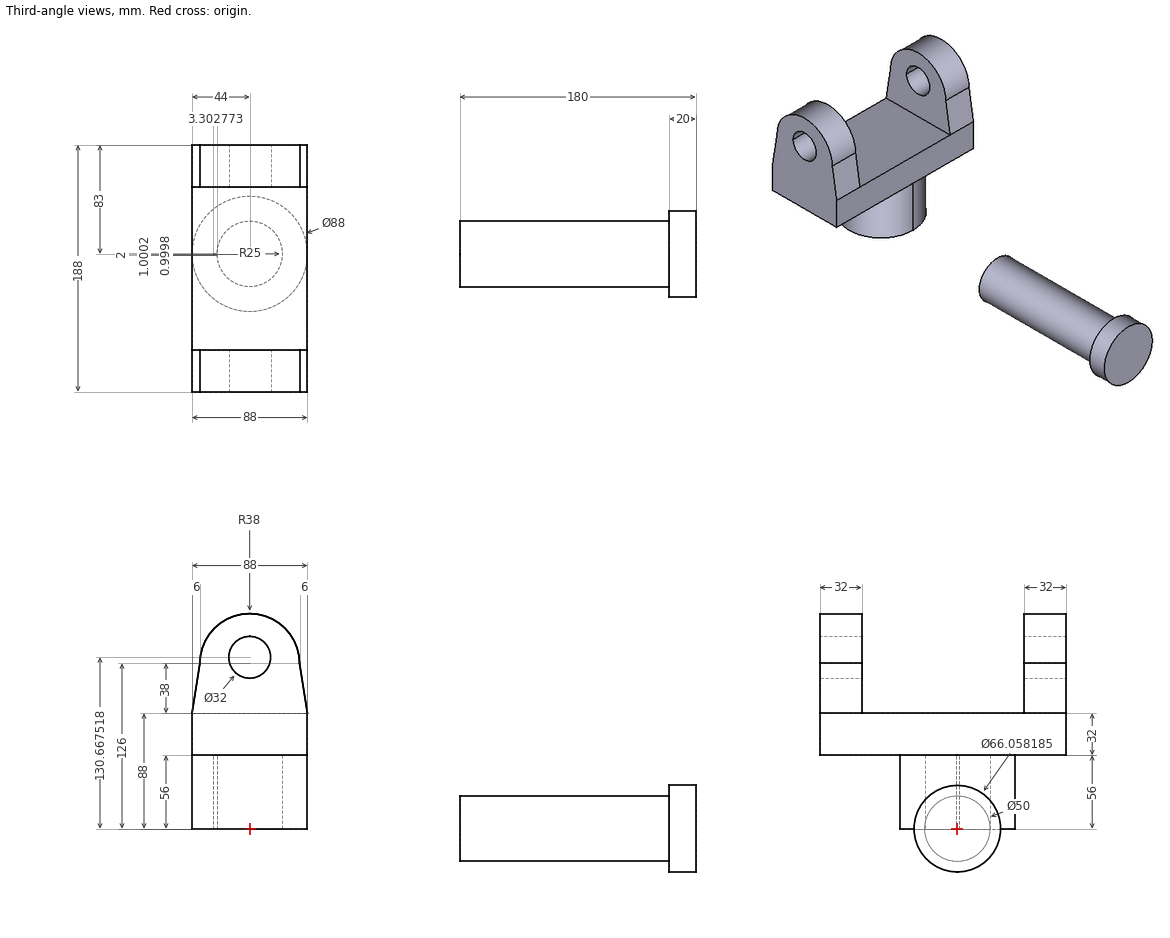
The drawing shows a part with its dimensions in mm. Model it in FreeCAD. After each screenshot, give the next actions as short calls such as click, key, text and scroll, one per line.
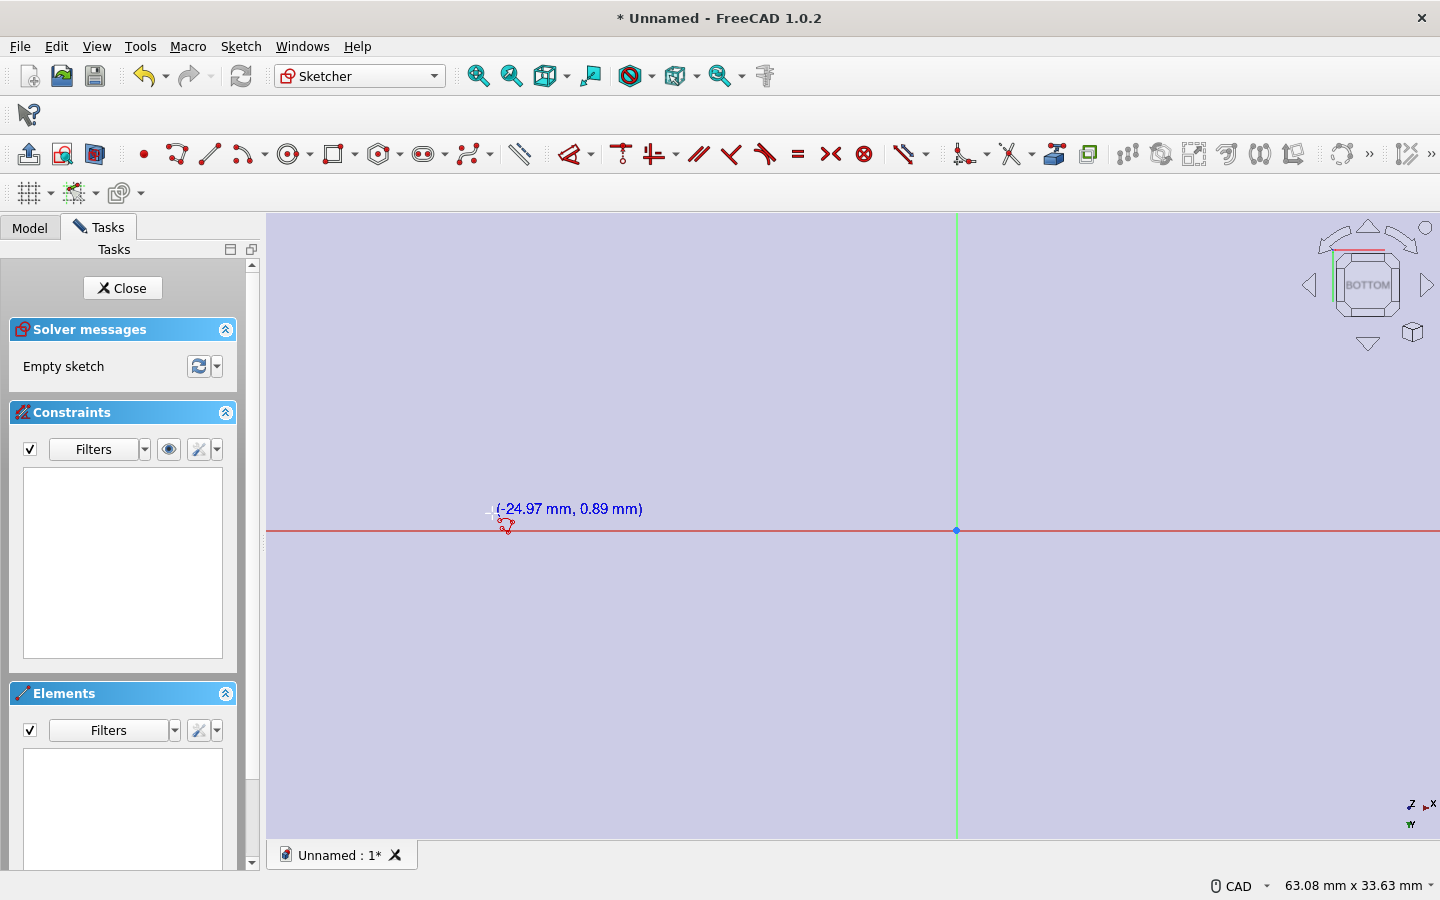
click(492, 512)
click(430, 508)
click(430, 549)
click(492, 549)
right_click(492, 549)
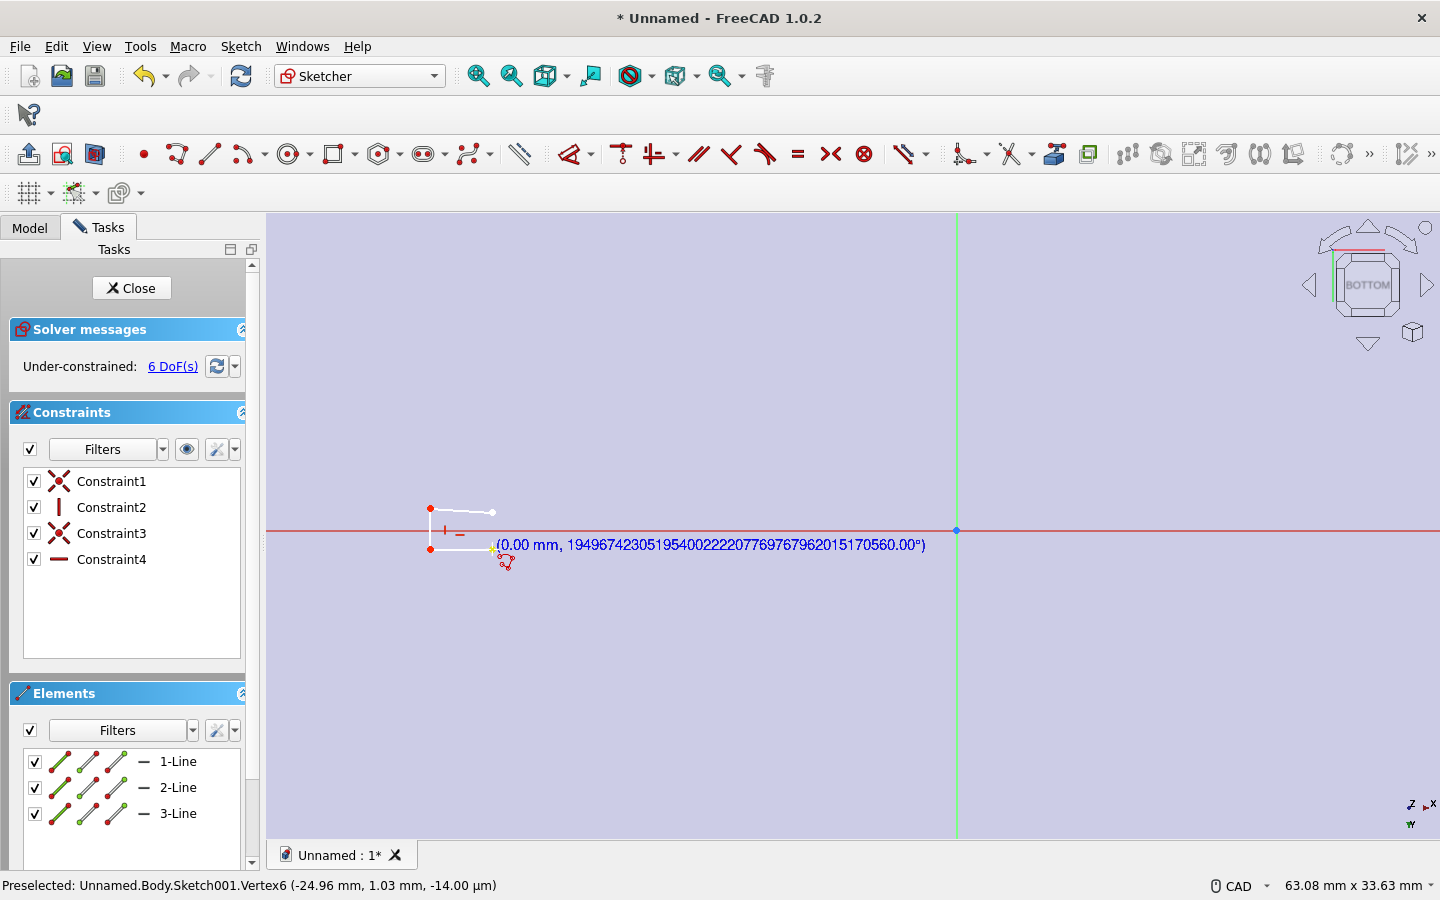
key(g)
key(3)
key(a)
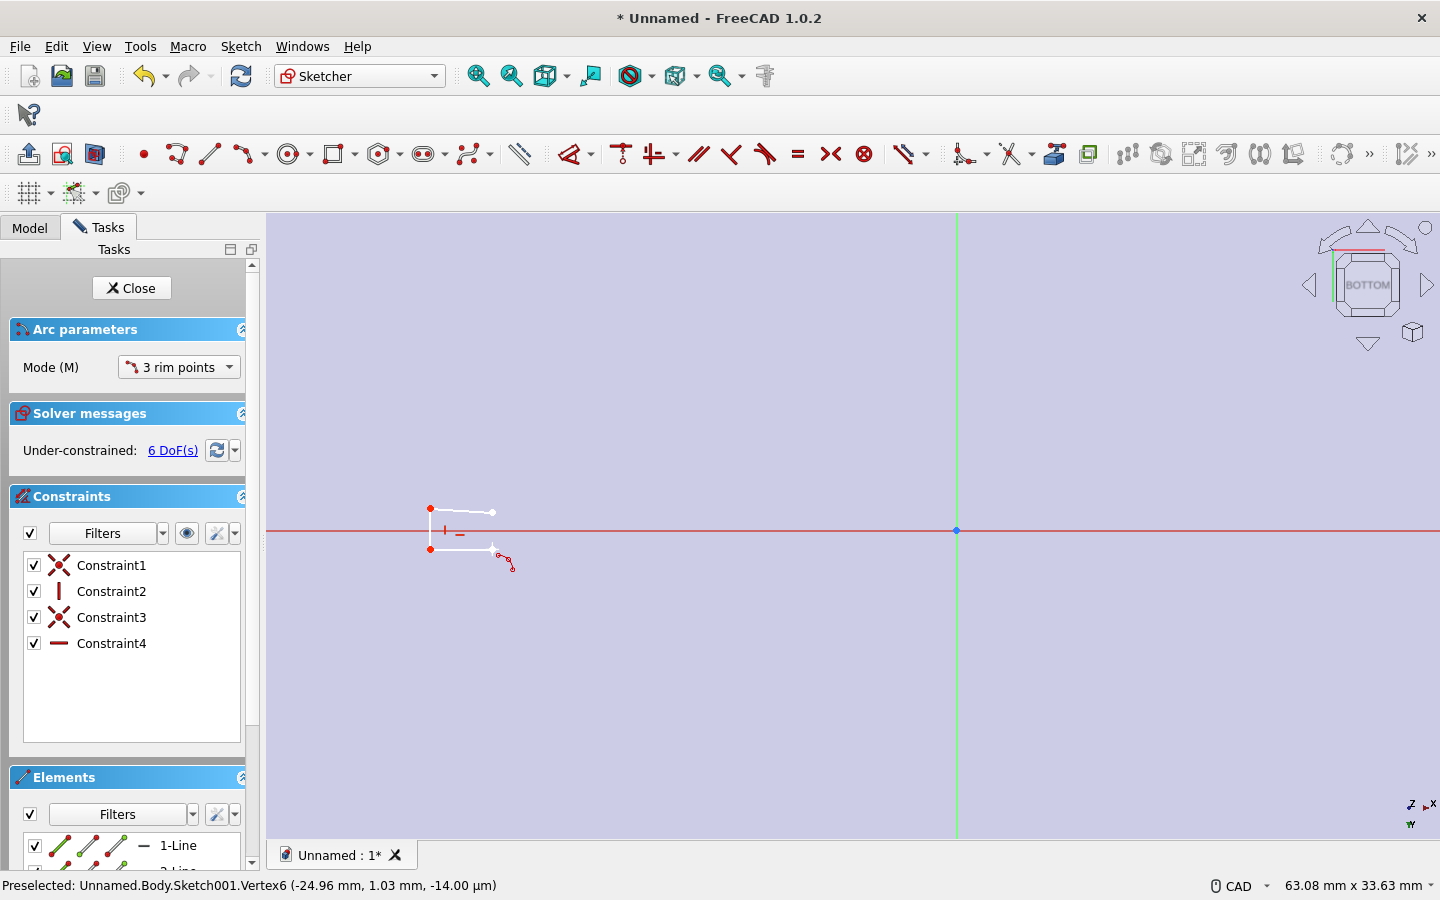
click(492, 550)
click(492, 513)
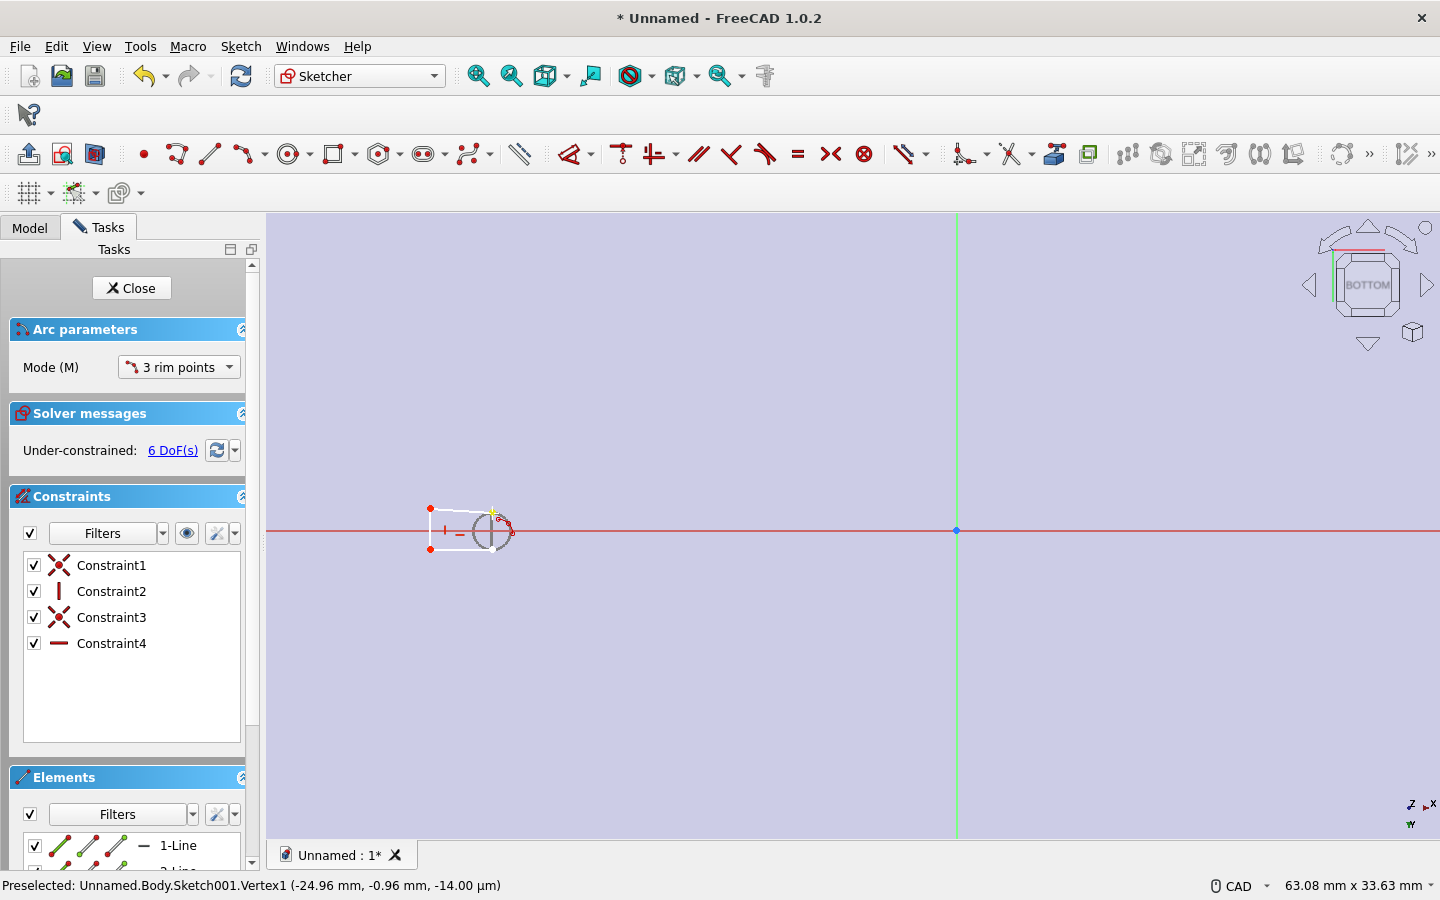
scroll(497, 516, down, 2)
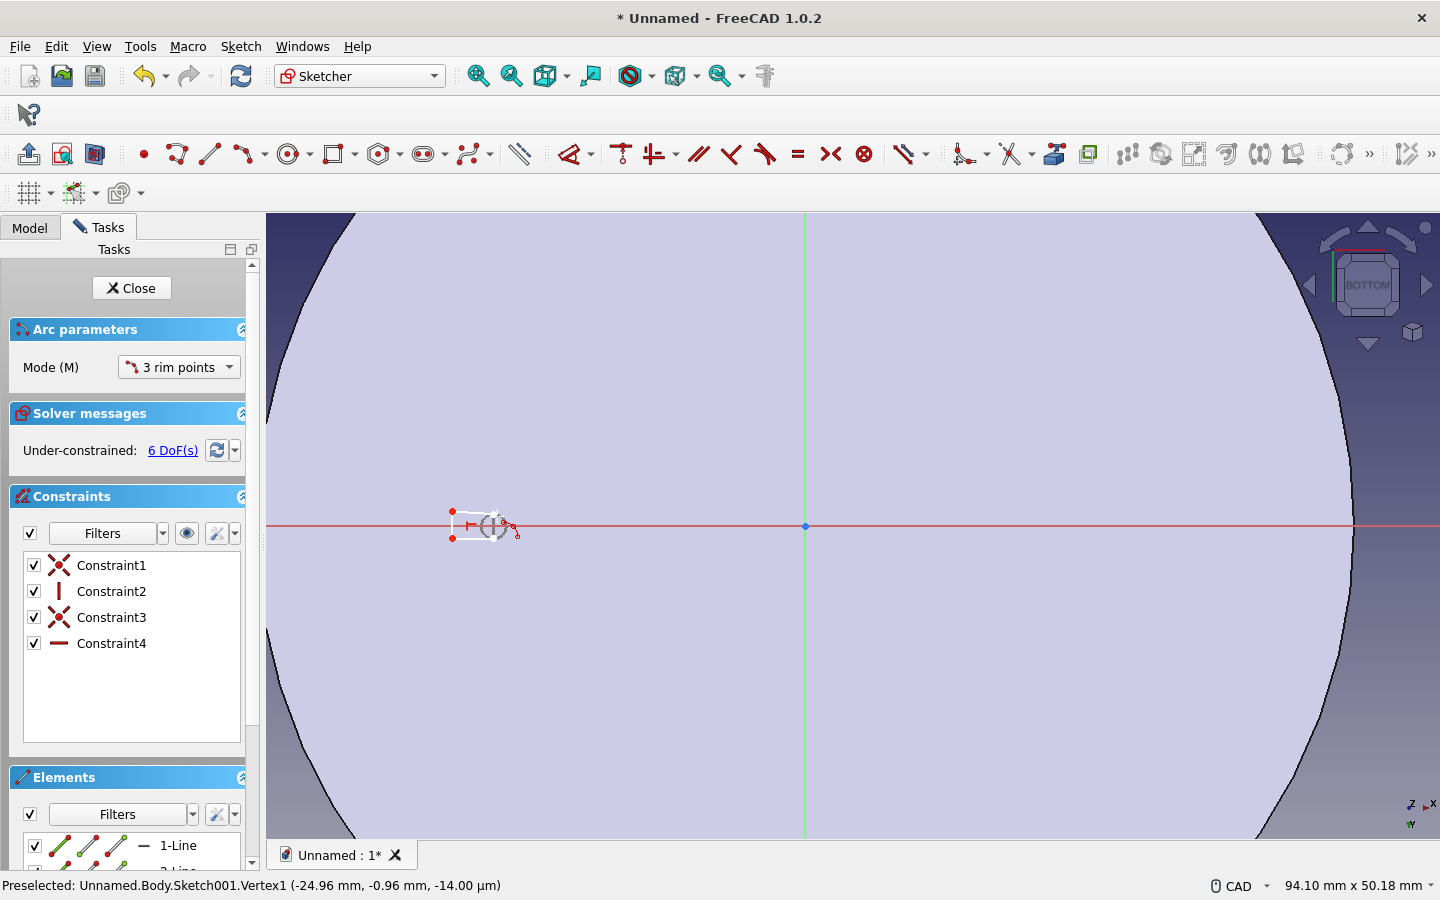
click(1059, 707)
key(Escape)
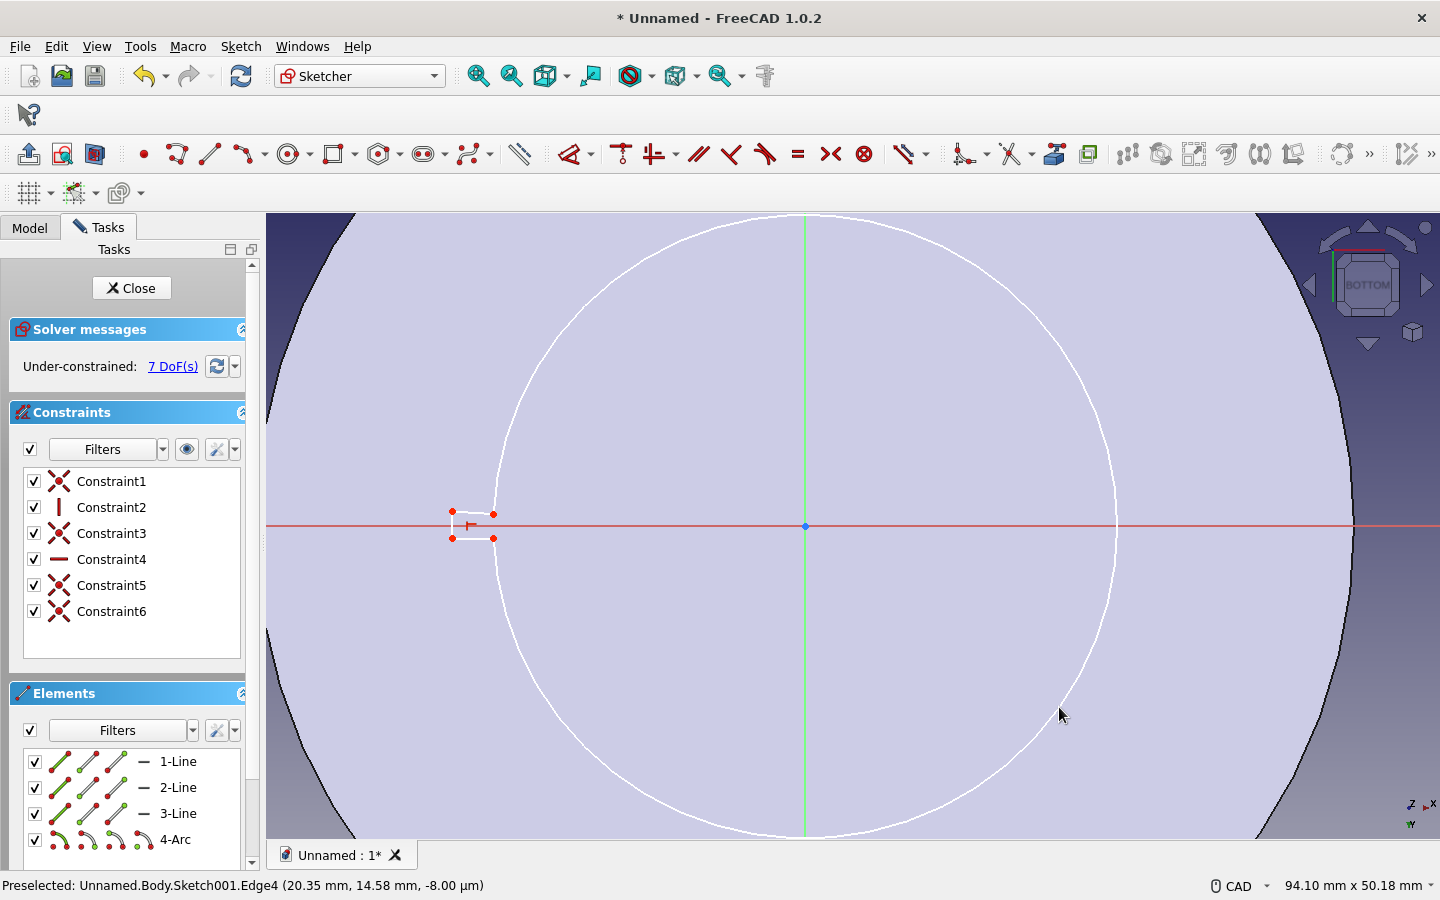
drag(795, 516, 815, 537)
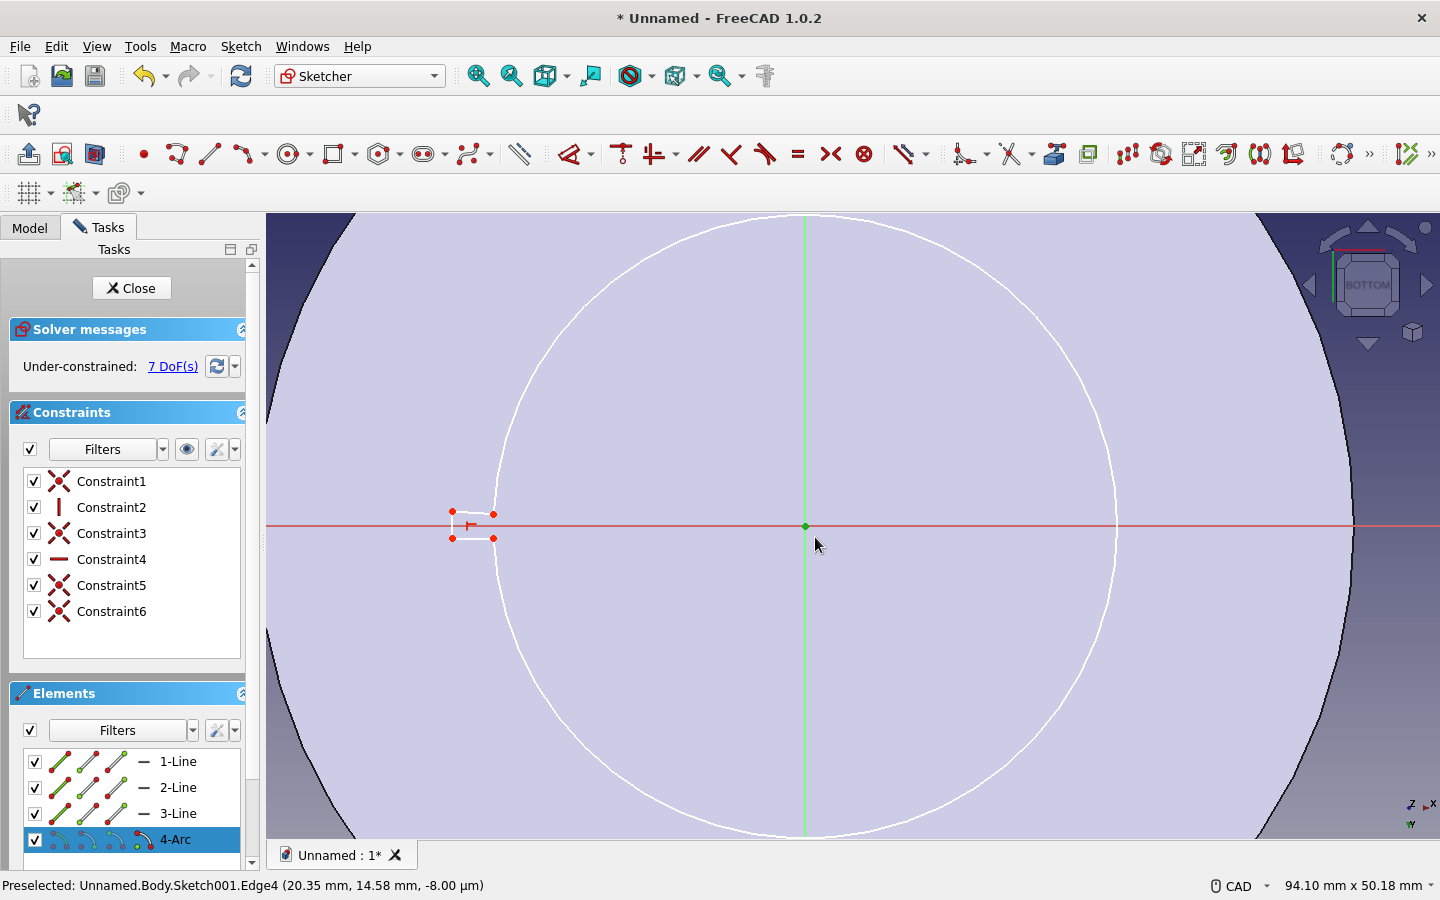
key(c)